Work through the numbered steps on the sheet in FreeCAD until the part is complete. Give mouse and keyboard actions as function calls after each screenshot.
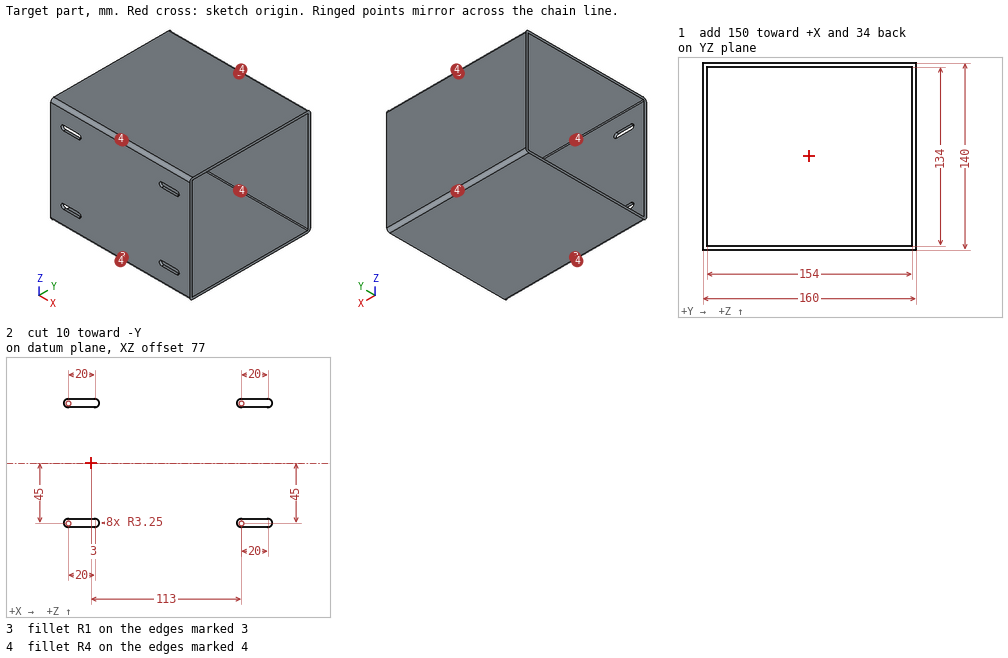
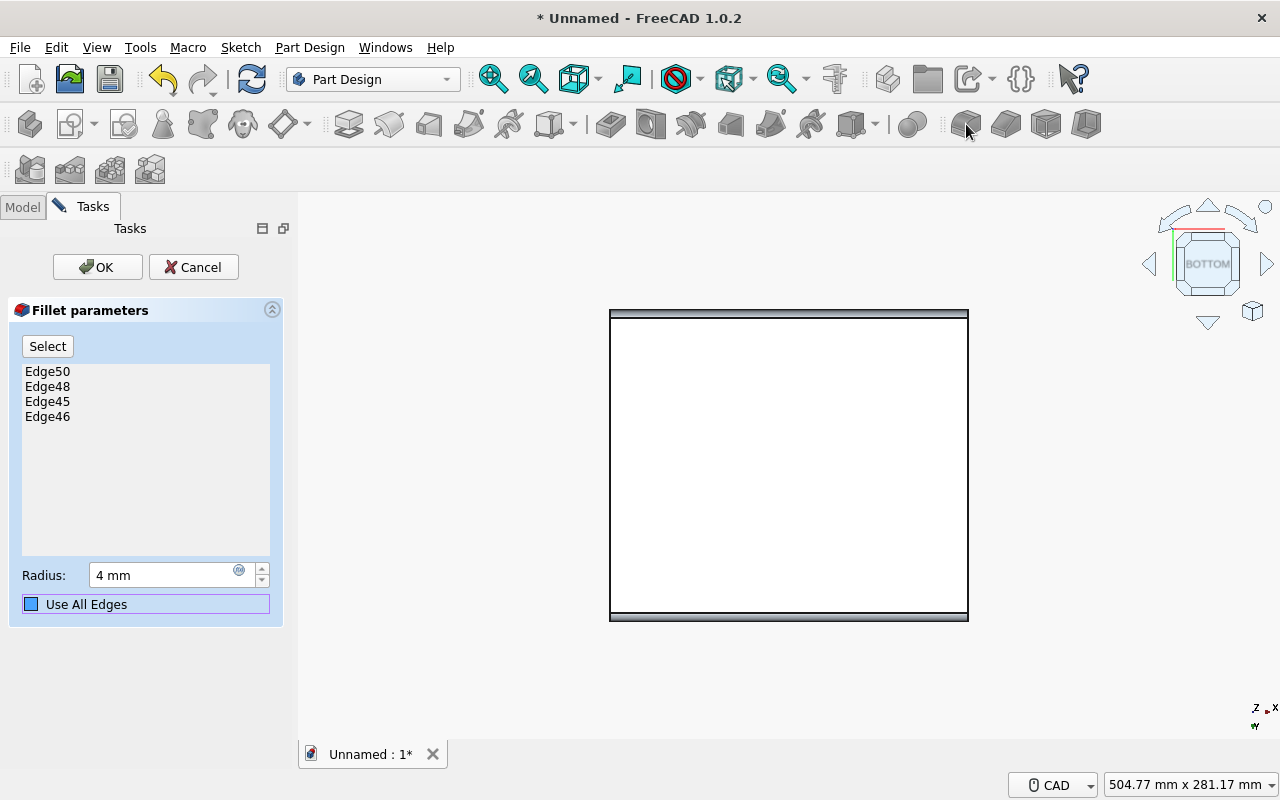
click(98, 267)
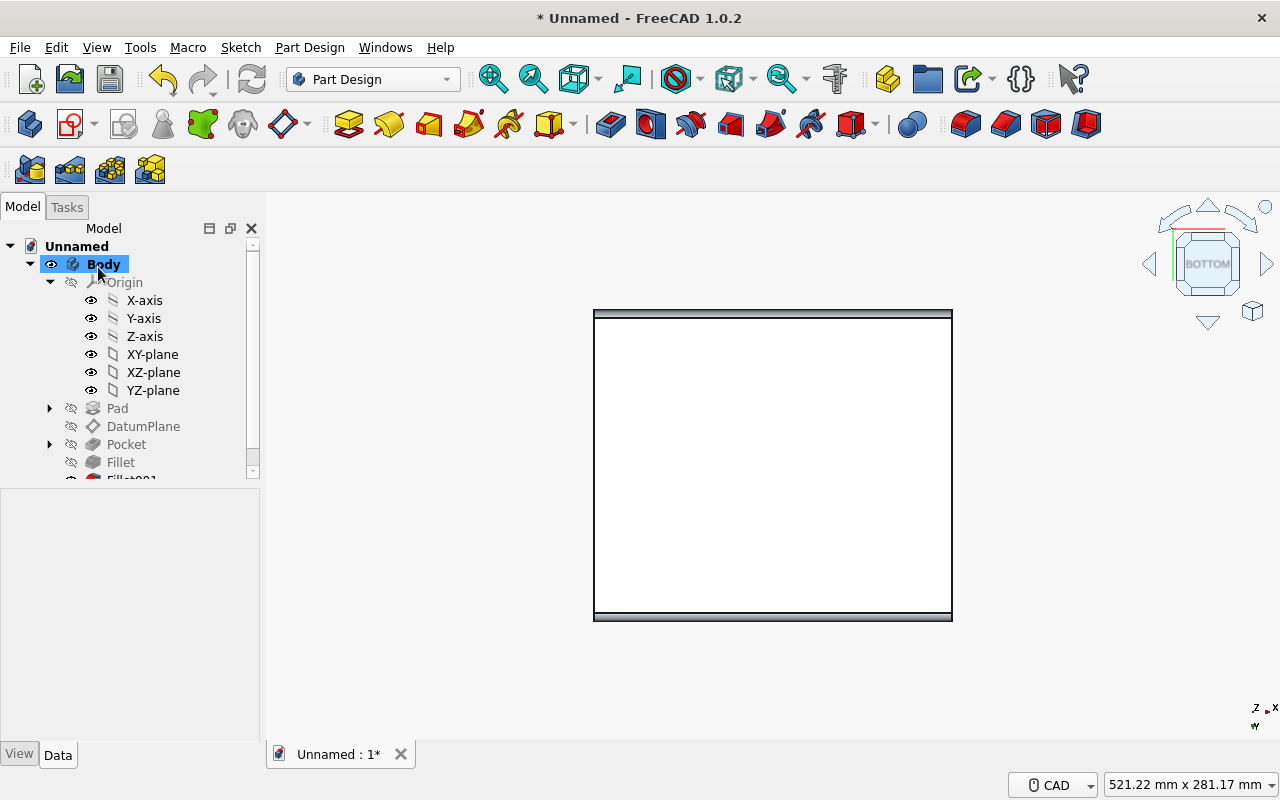
key(0)